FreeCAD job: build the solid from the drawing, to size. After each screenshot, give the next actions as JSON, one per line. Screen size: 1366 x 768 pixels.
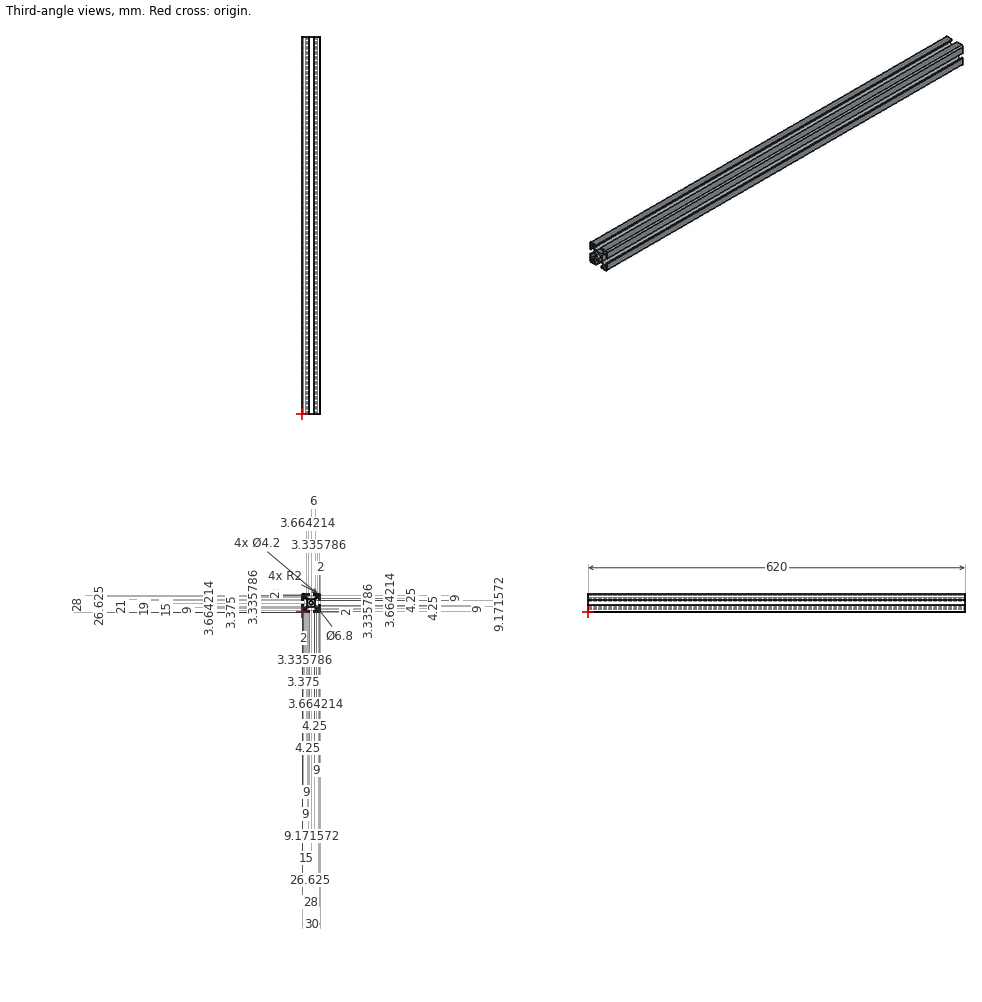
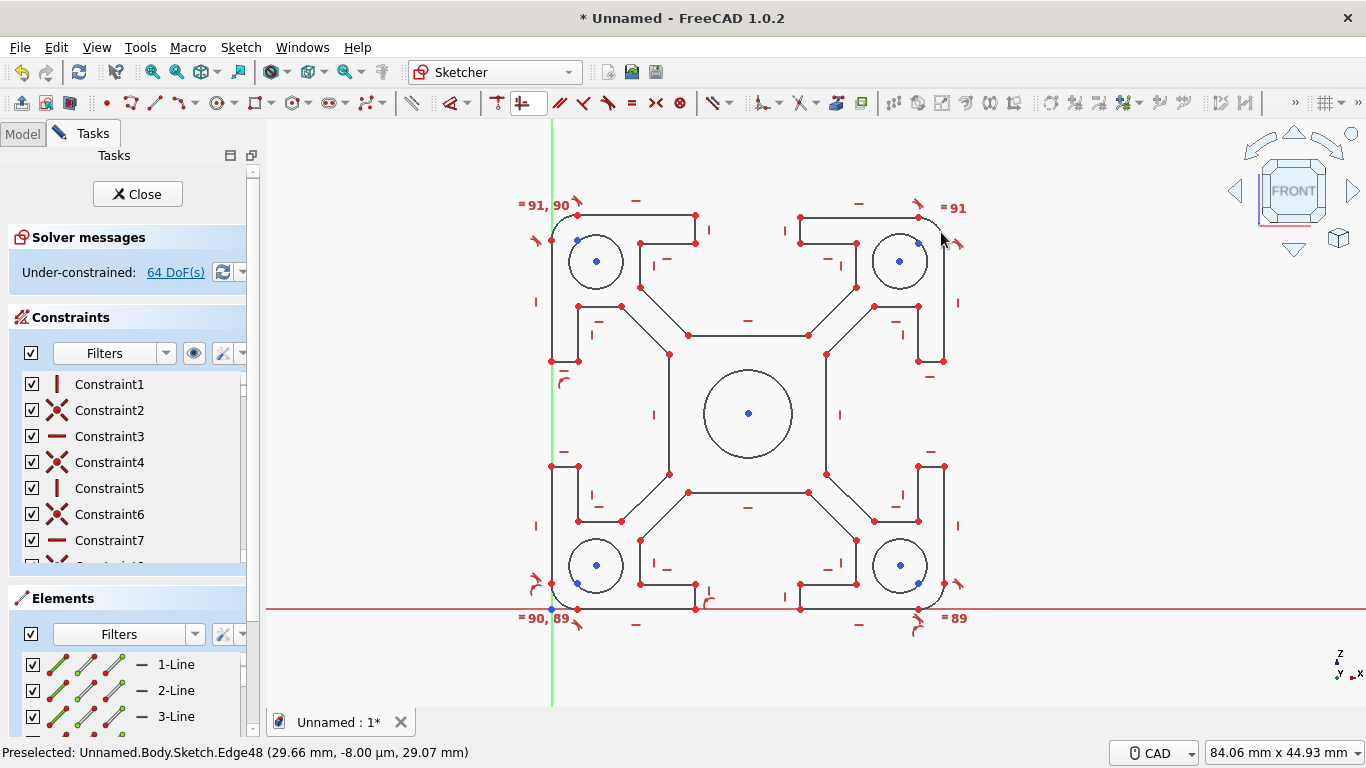
{"action": "left_click", "coordinate": [881, 242]}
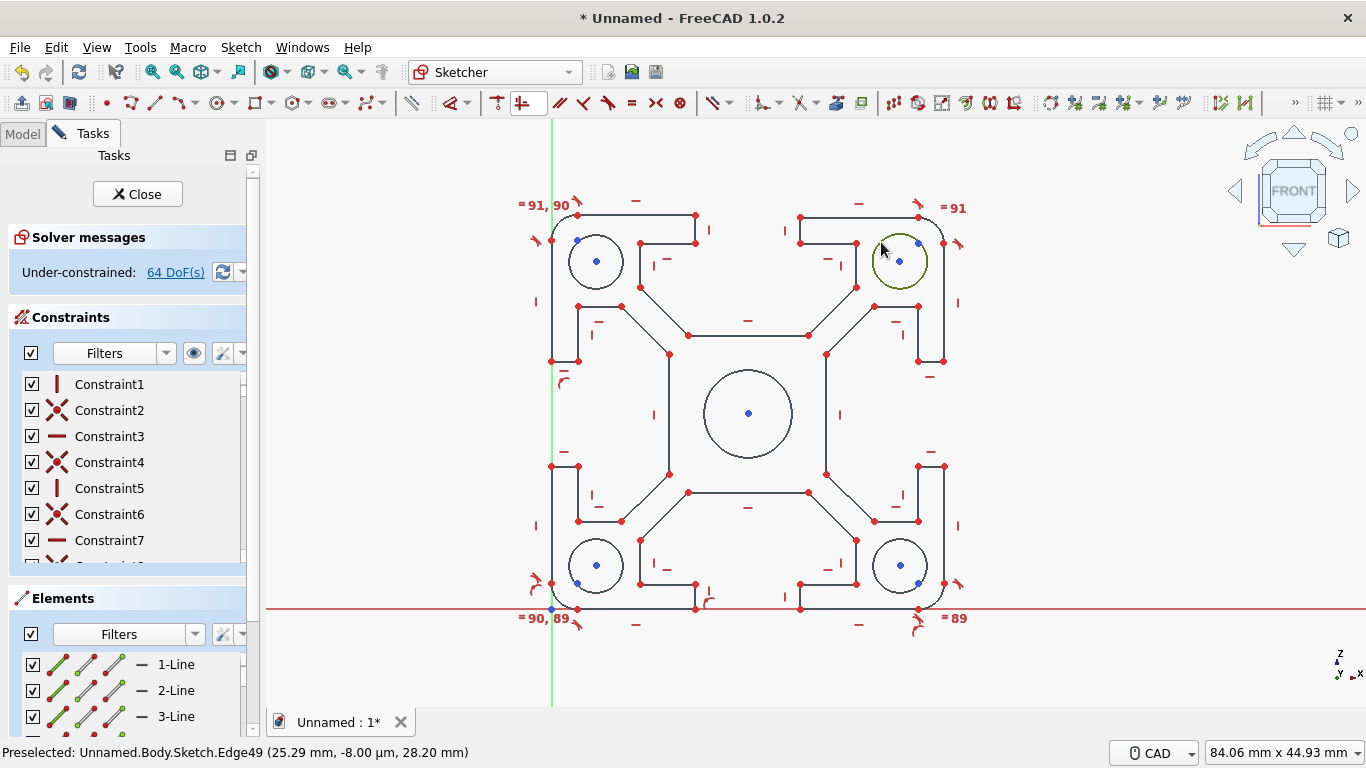
{"action": "left_click", "coordinate": [615, 243]}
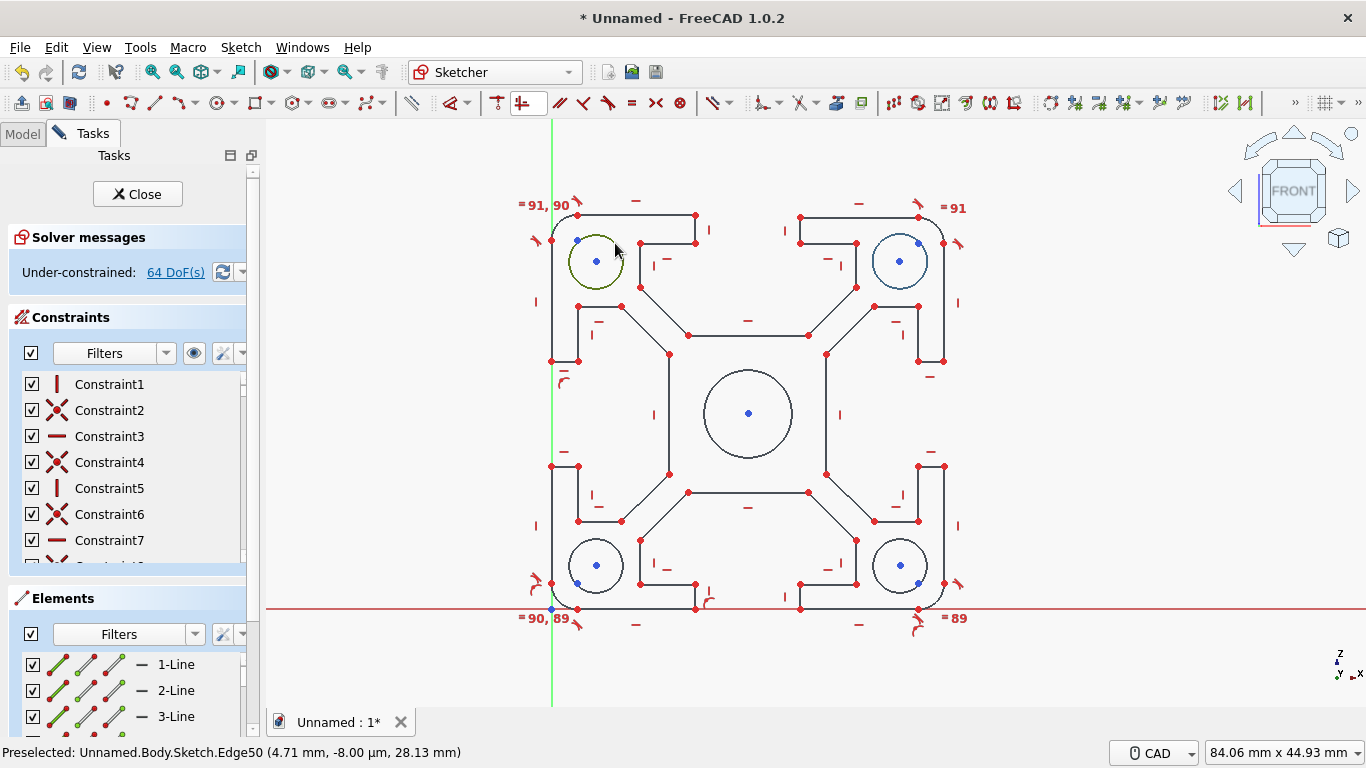
{"action": "left_click", "coordinate": [919, 547]}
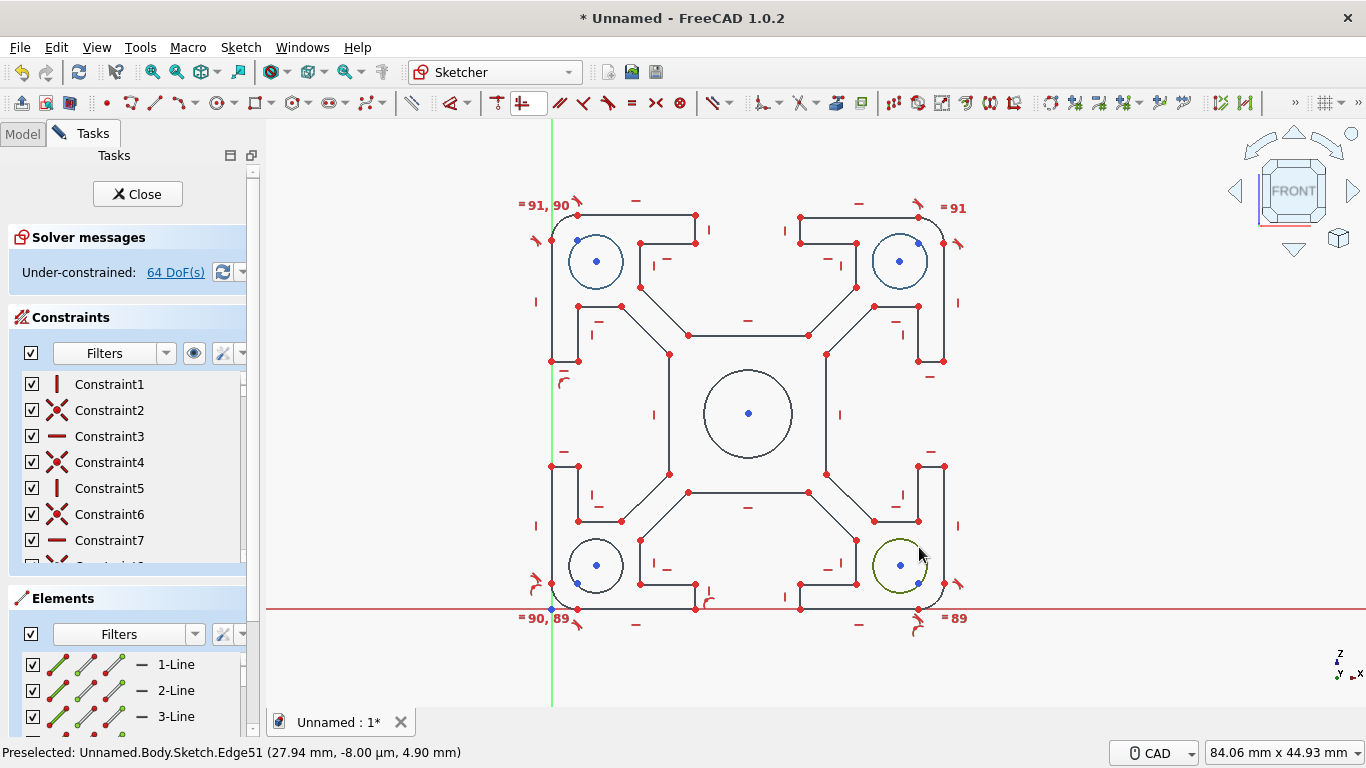
{"action": "left_click", "coordinate": [615, 547]}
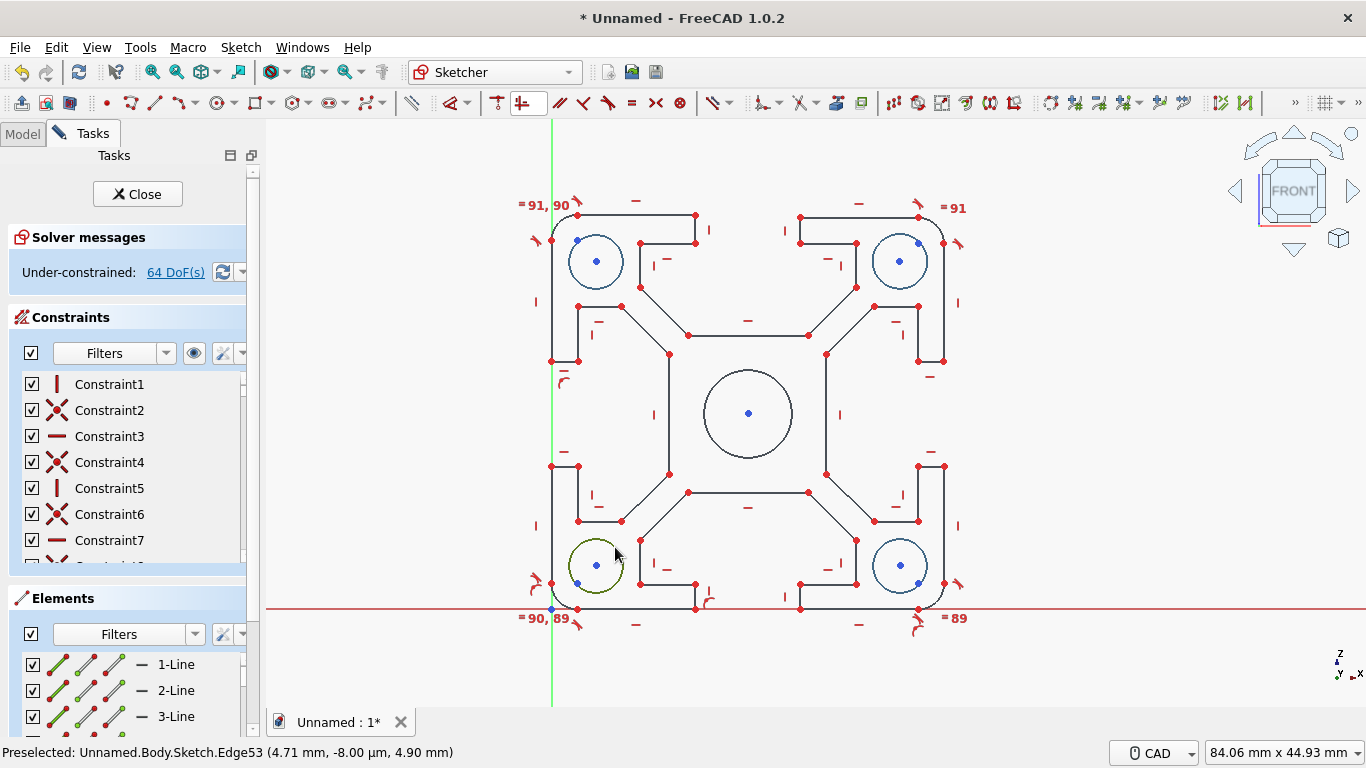
{"action": "key", "text": "e"}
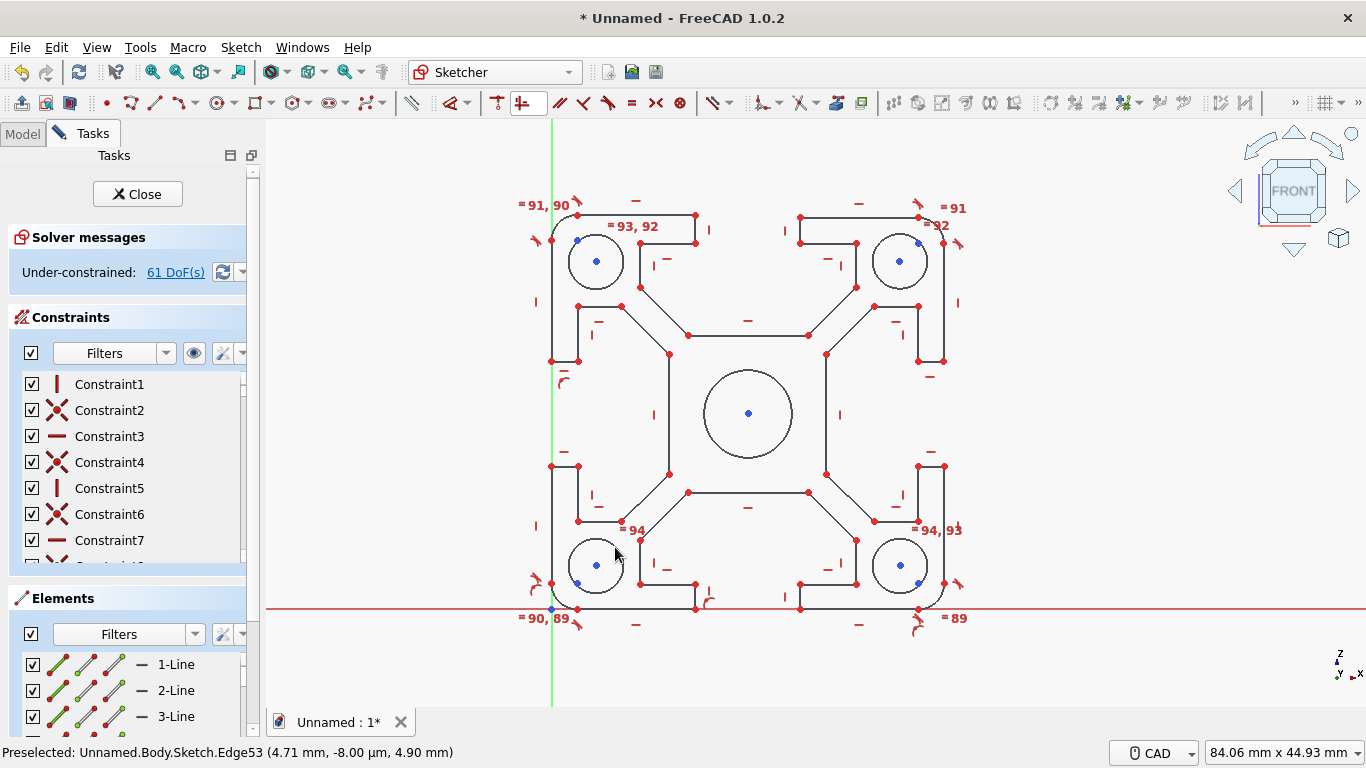
{"action": "key", "text": "d"}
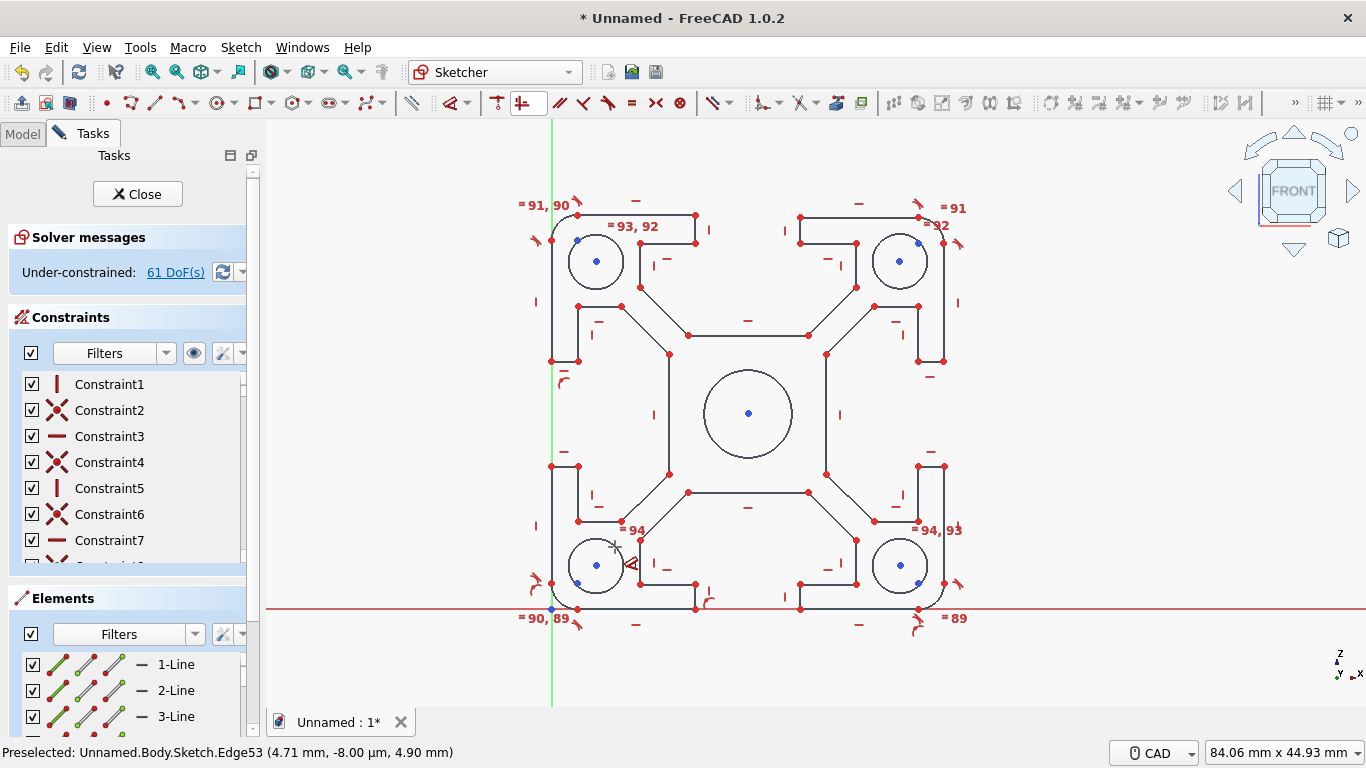
{"action": "scroll", "coordinate": [930, 607], "scroll_direction": "up", "scroll_amount": 3}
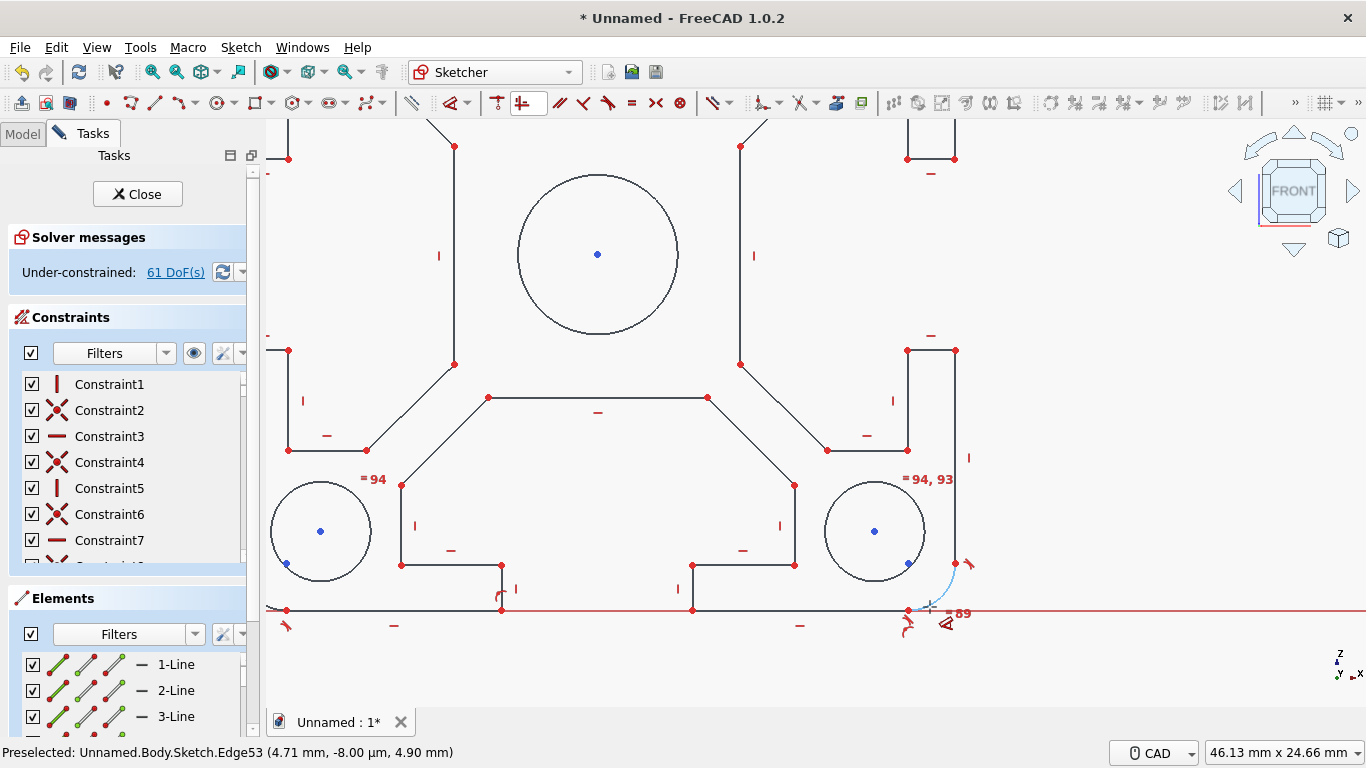
{"action": "left_click", "coordinate": [929, 605]}
{"action": "left_click", "coordinate": [943, 634]}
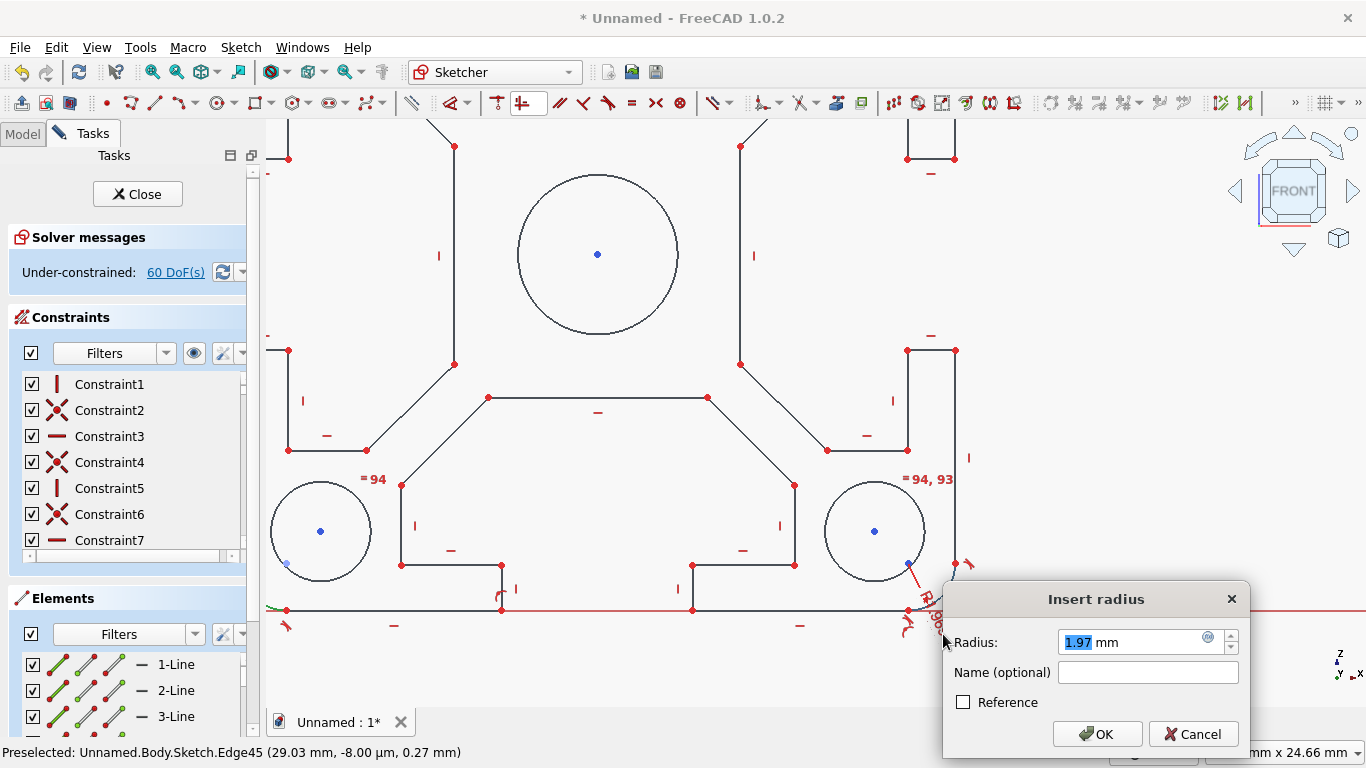
{"action": "type", "text": "2"}
{"action": "key", "text": "Return"}